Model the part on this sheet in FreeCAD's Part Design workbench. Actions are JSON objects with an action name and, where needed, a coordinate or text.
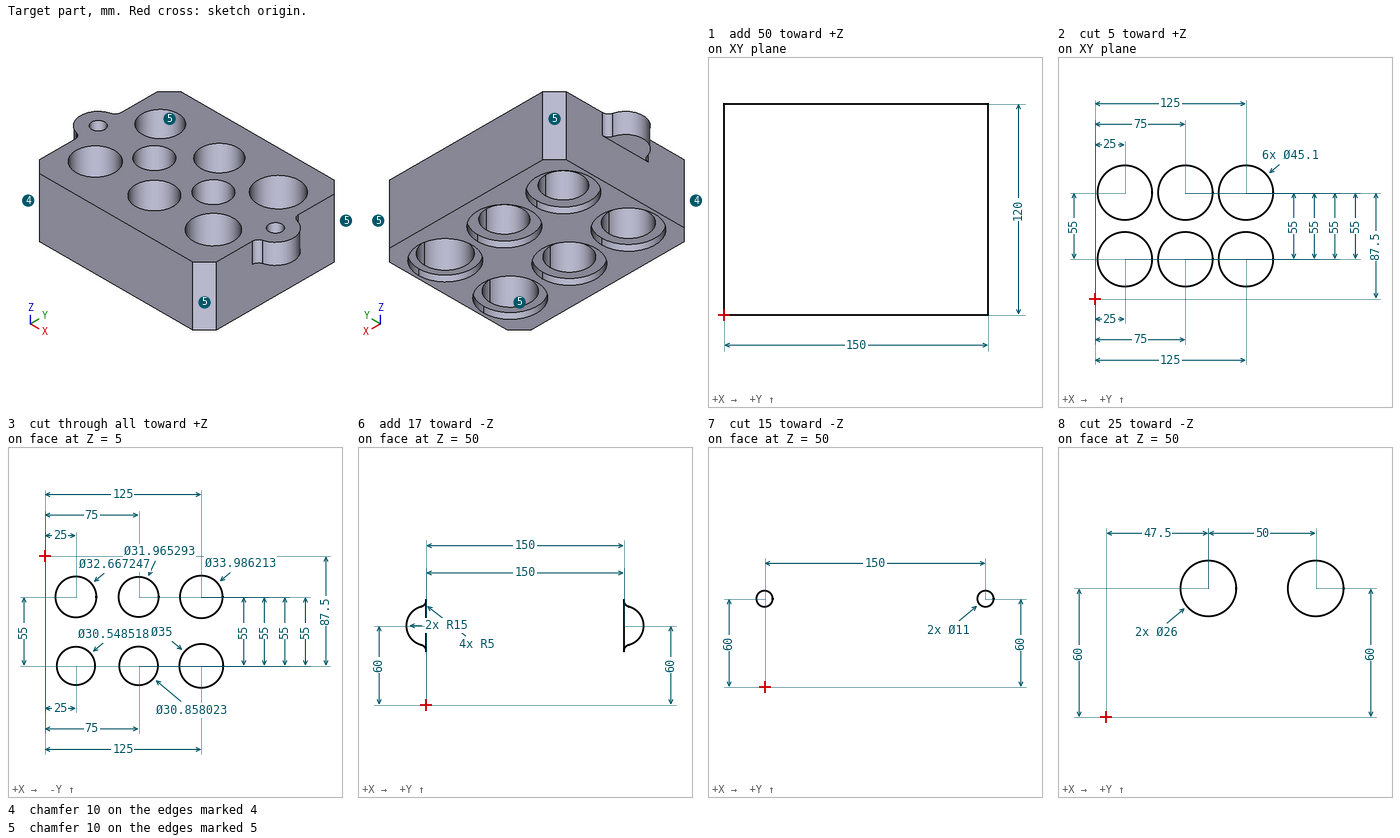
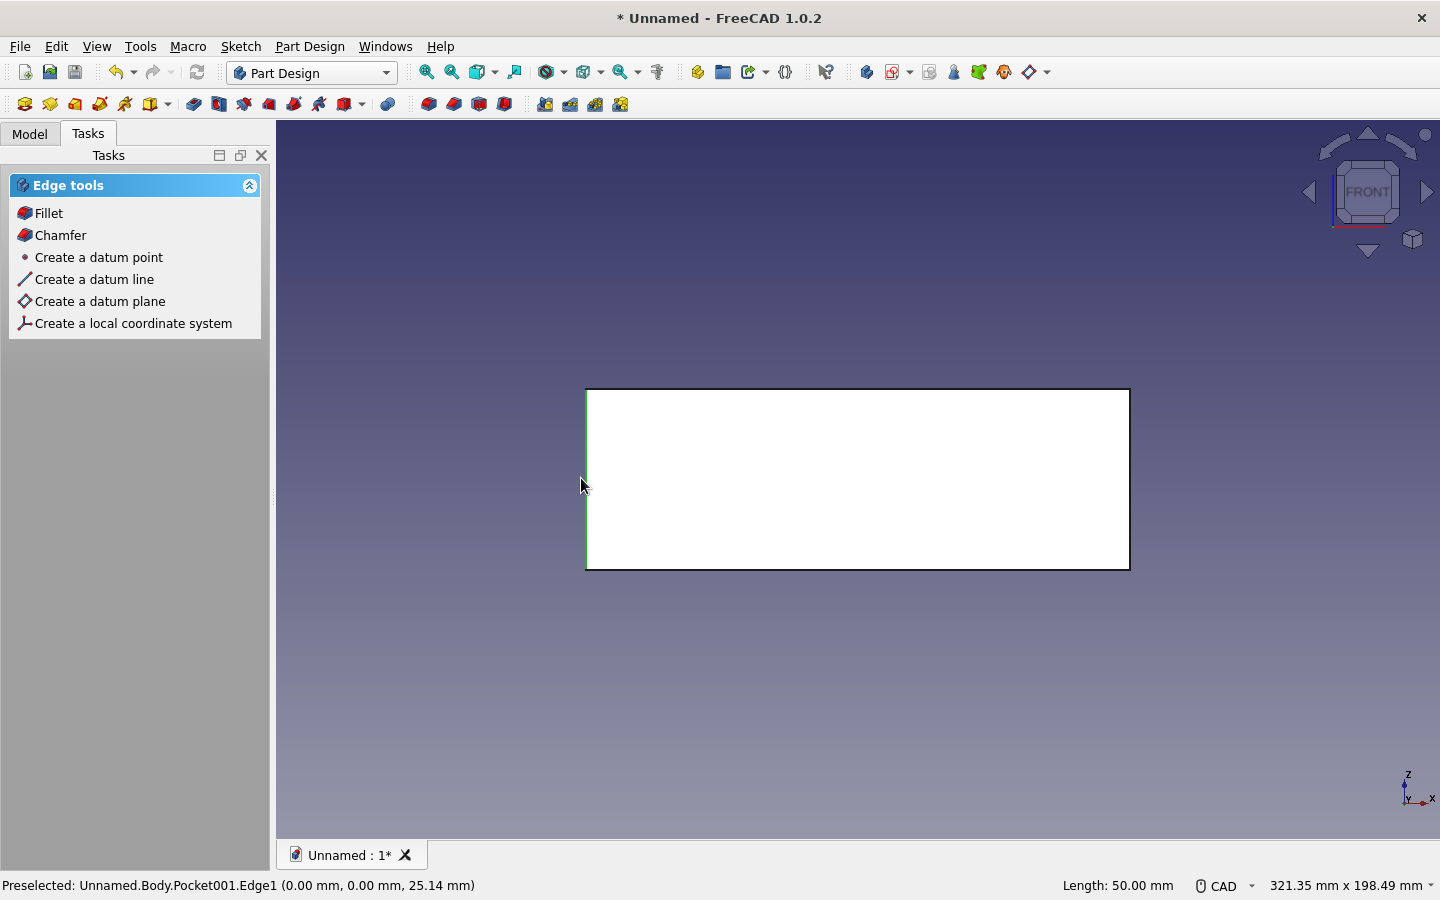
{"action": "left_click", "coordinate": [454, 104]}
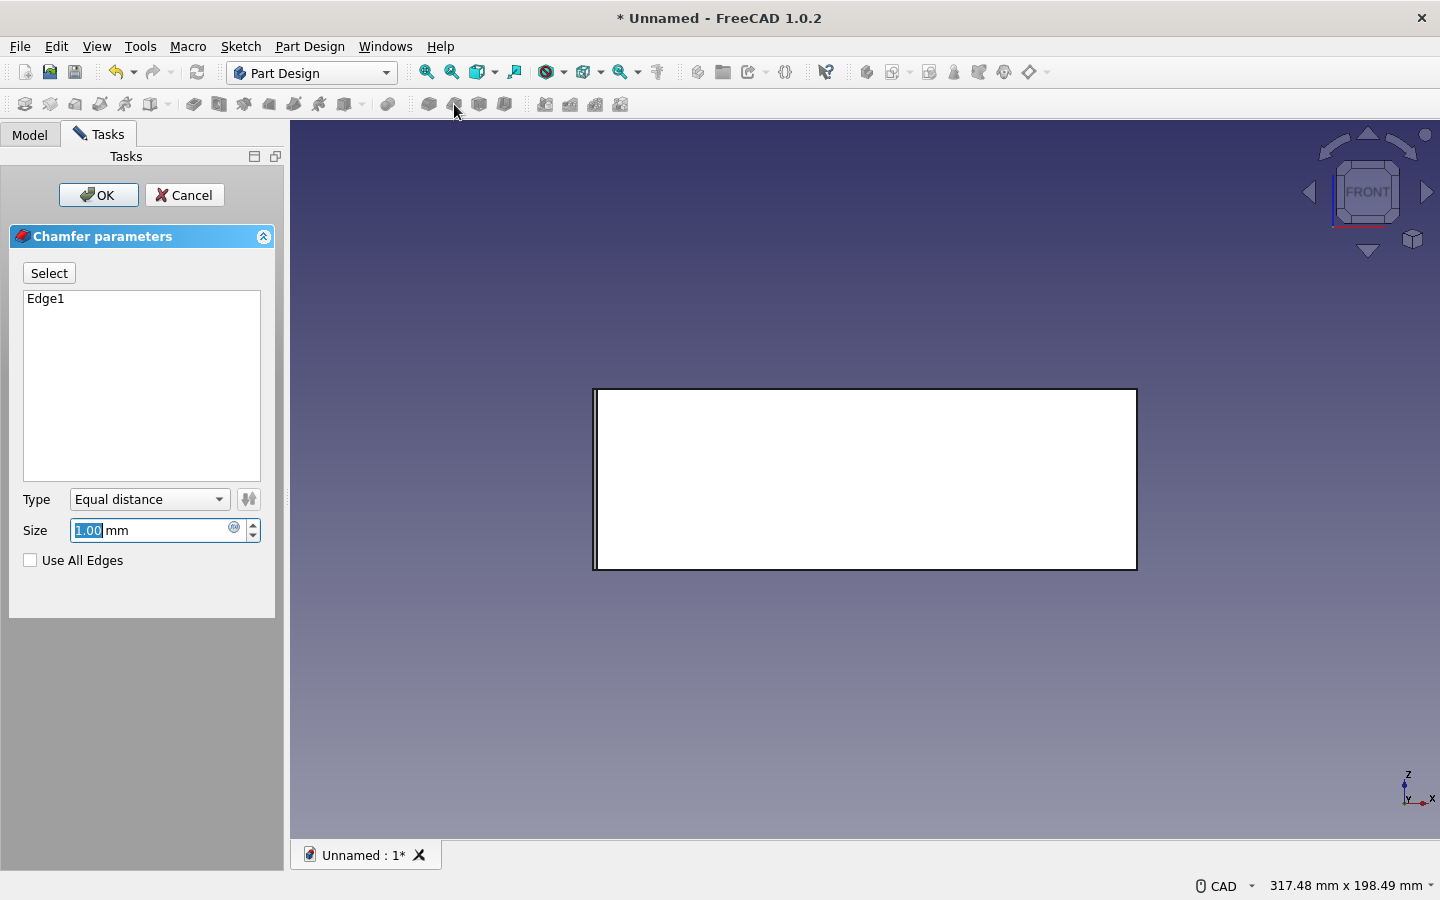
{"action": "type", "text": "10"}
{"action": "key", "text": "Tab"}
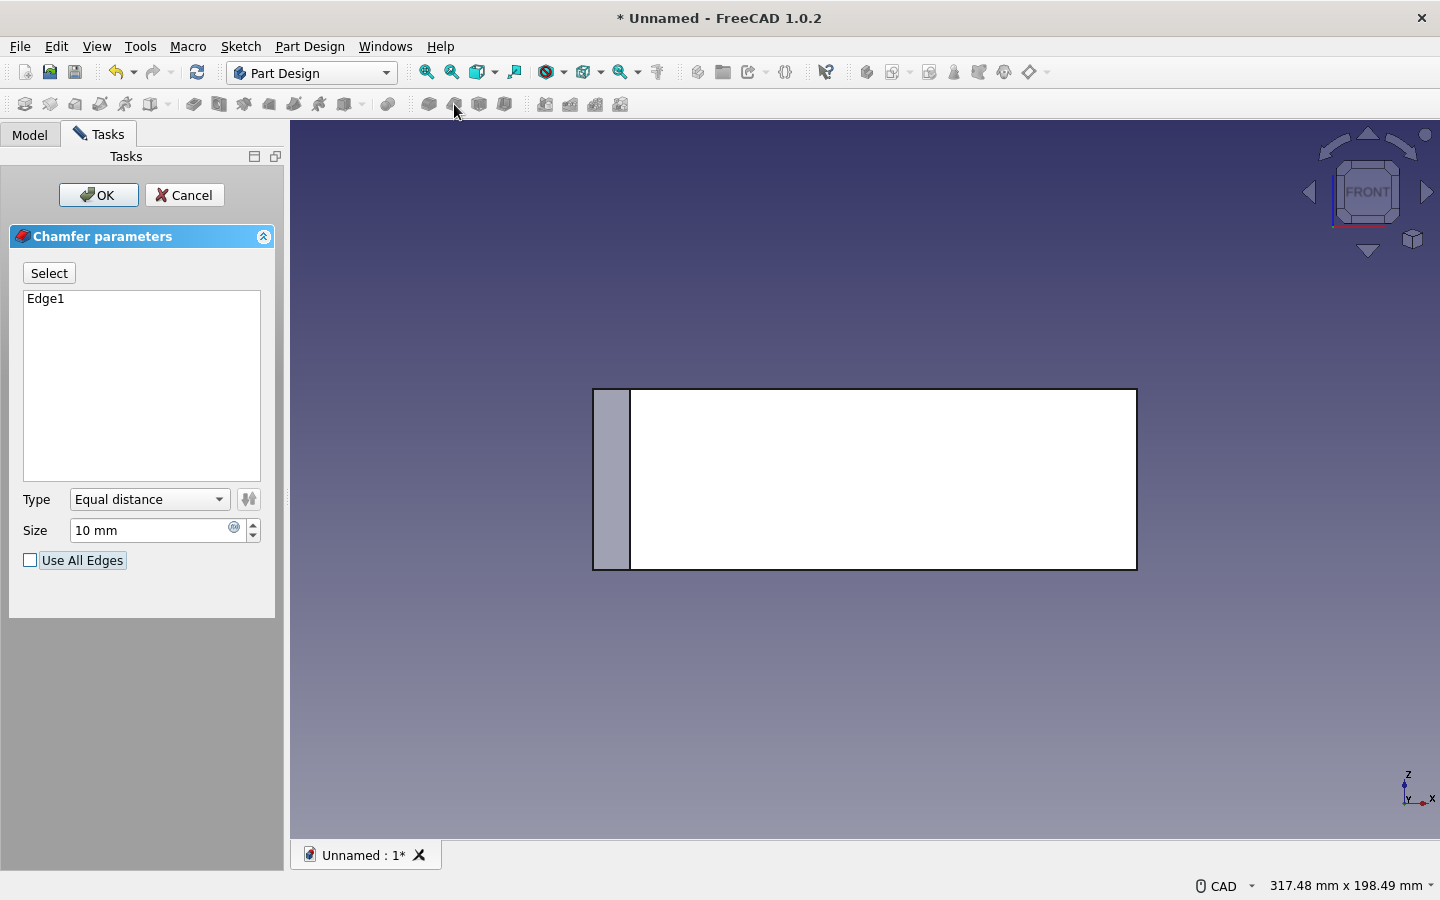
{"action": "left_click", "coordinate": [99, 195]}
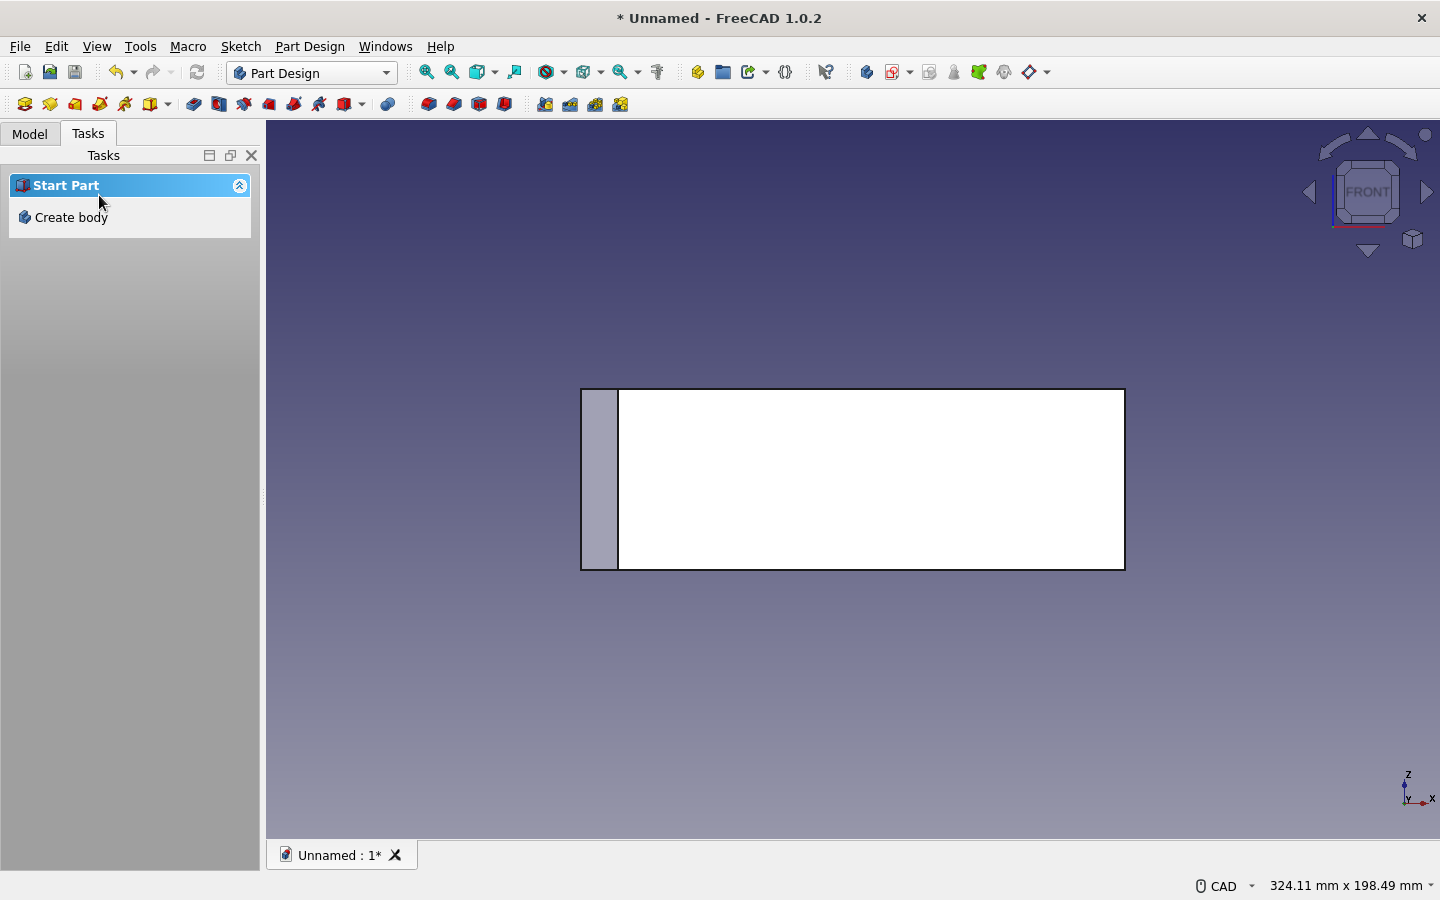
{"action": "left_click", "coordinate": [1125, 497]}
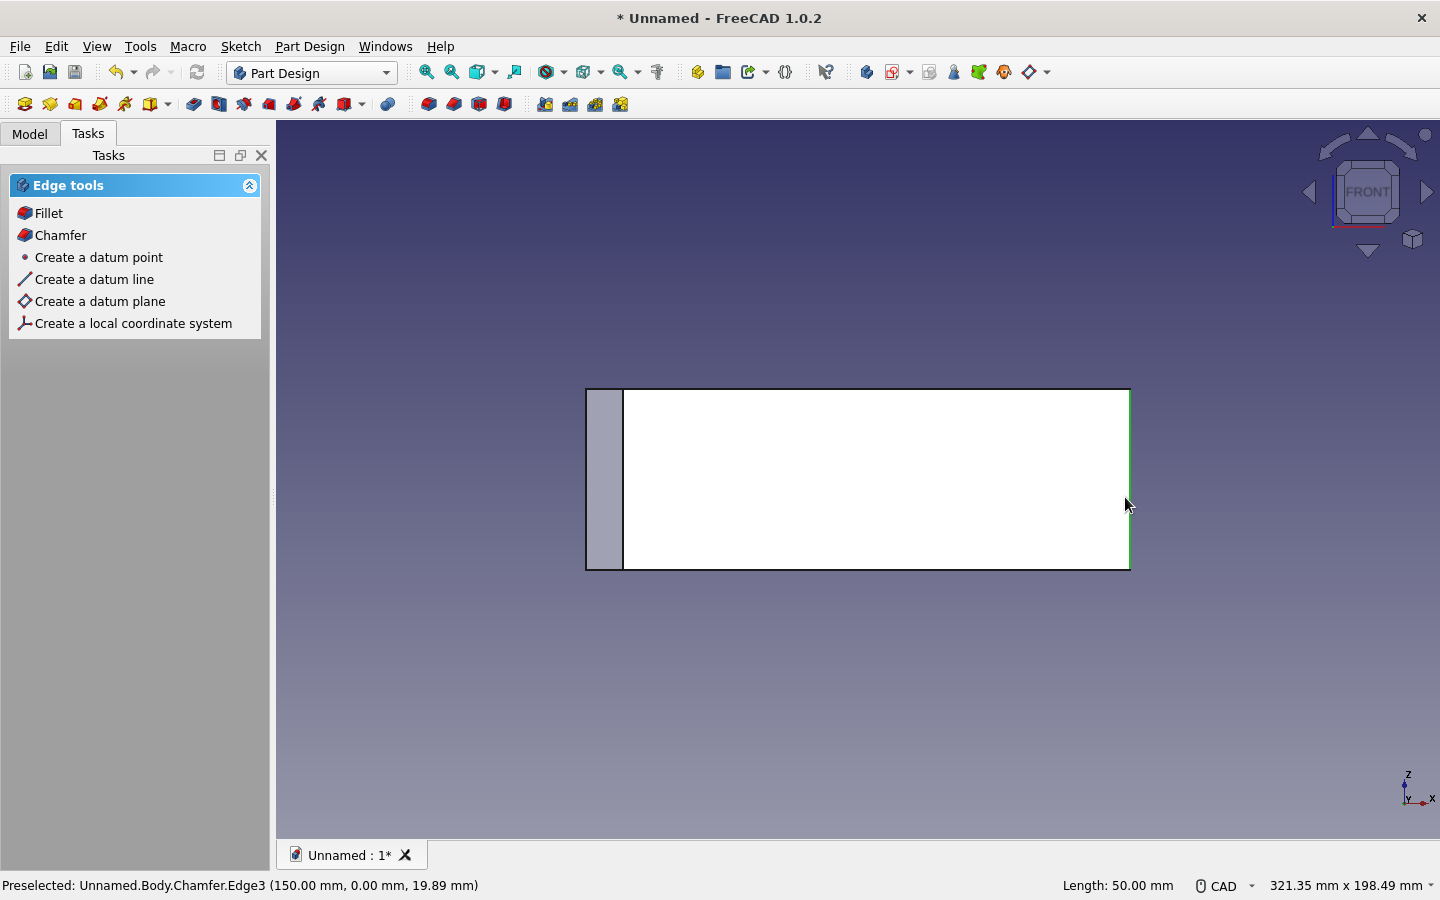
{"action": "key", "text": "0"}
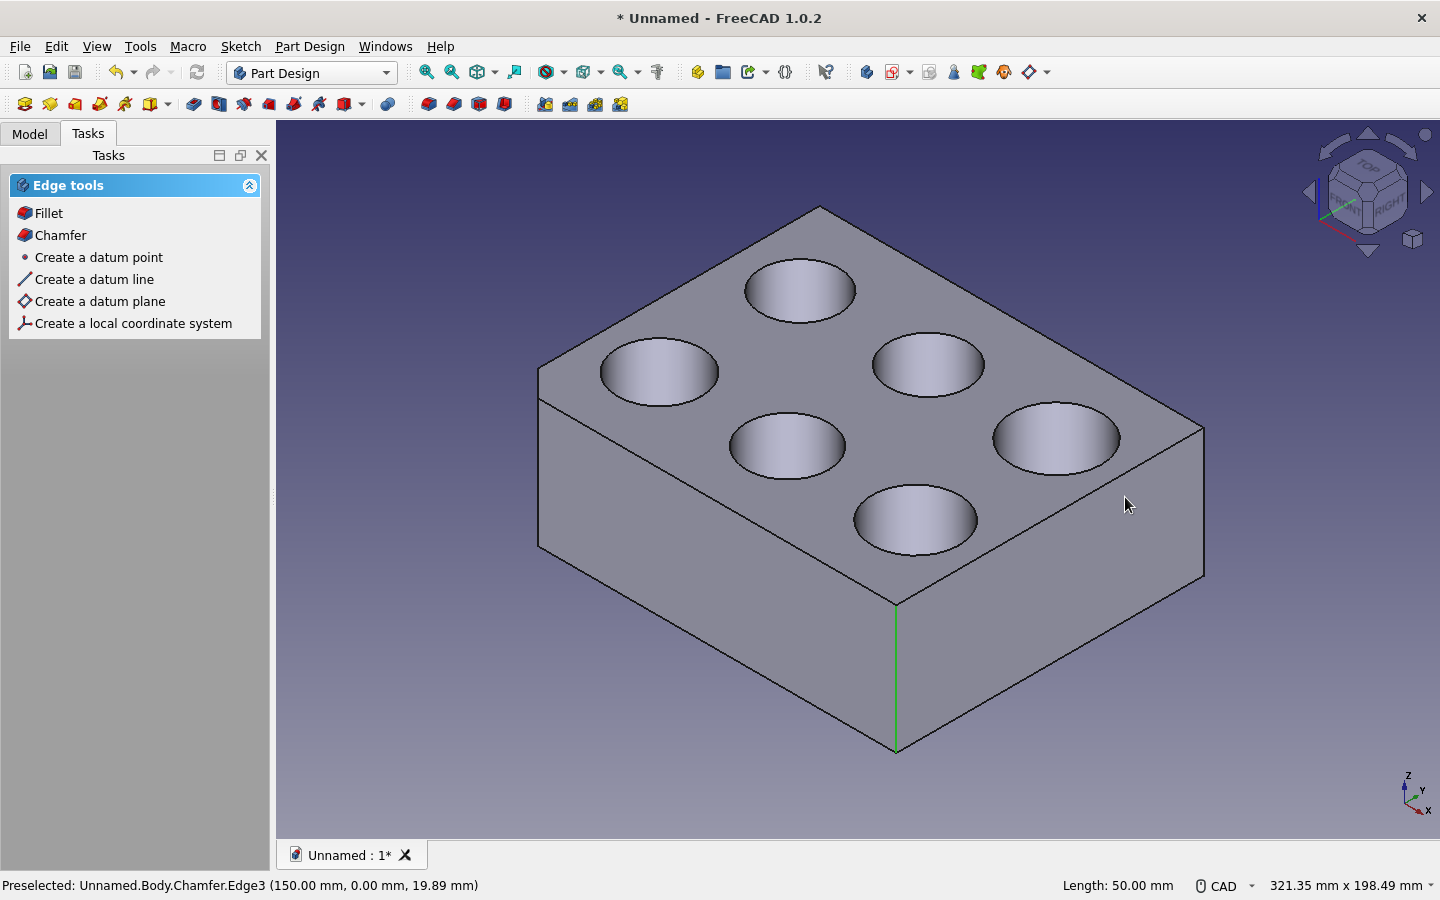
{"action": "key", "text": "2"}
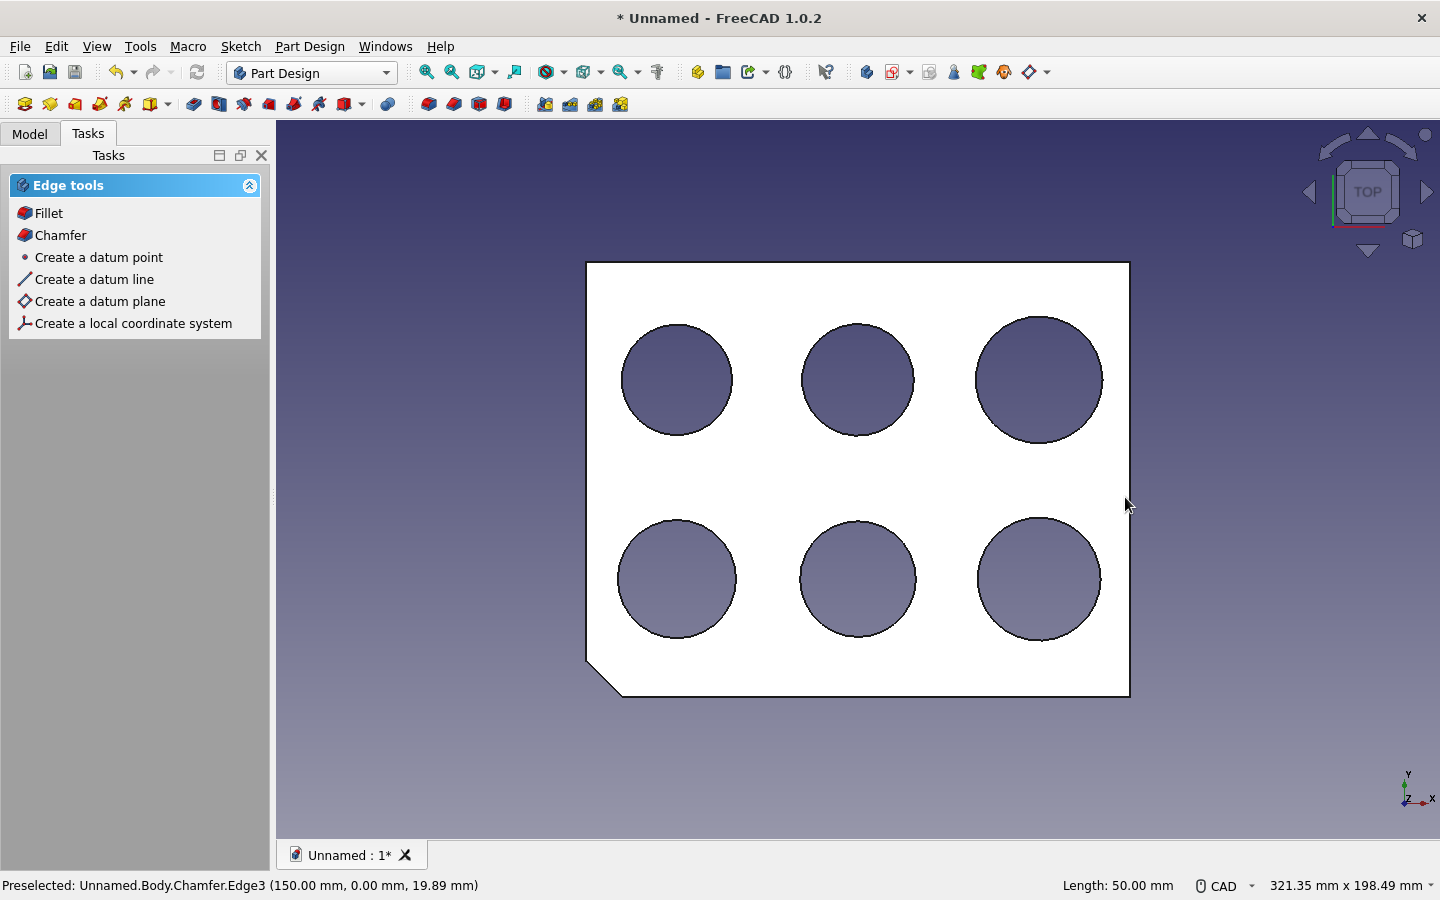
{"action": "key", "text": "1"}